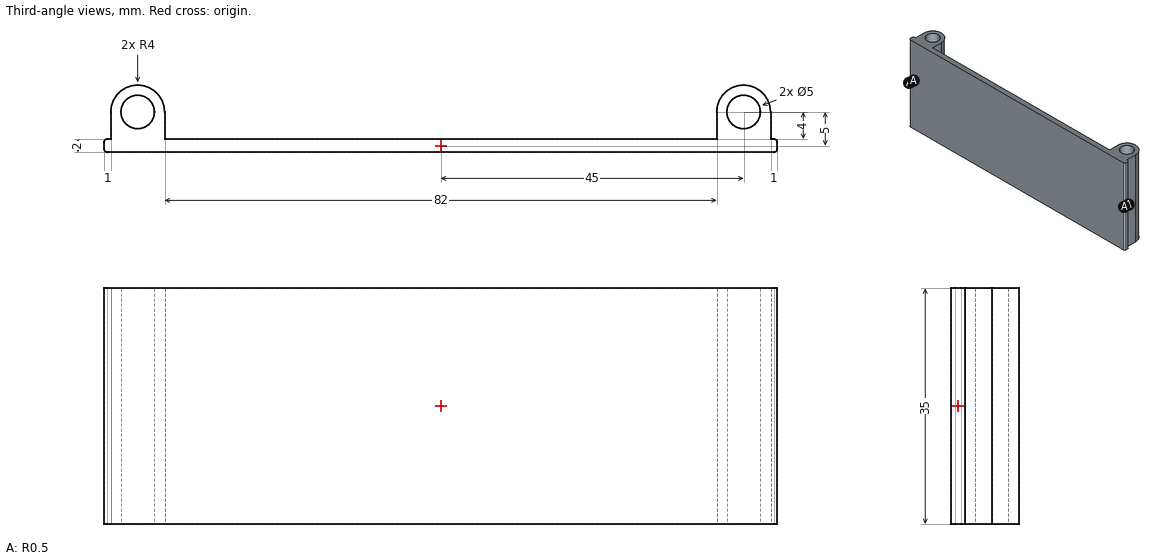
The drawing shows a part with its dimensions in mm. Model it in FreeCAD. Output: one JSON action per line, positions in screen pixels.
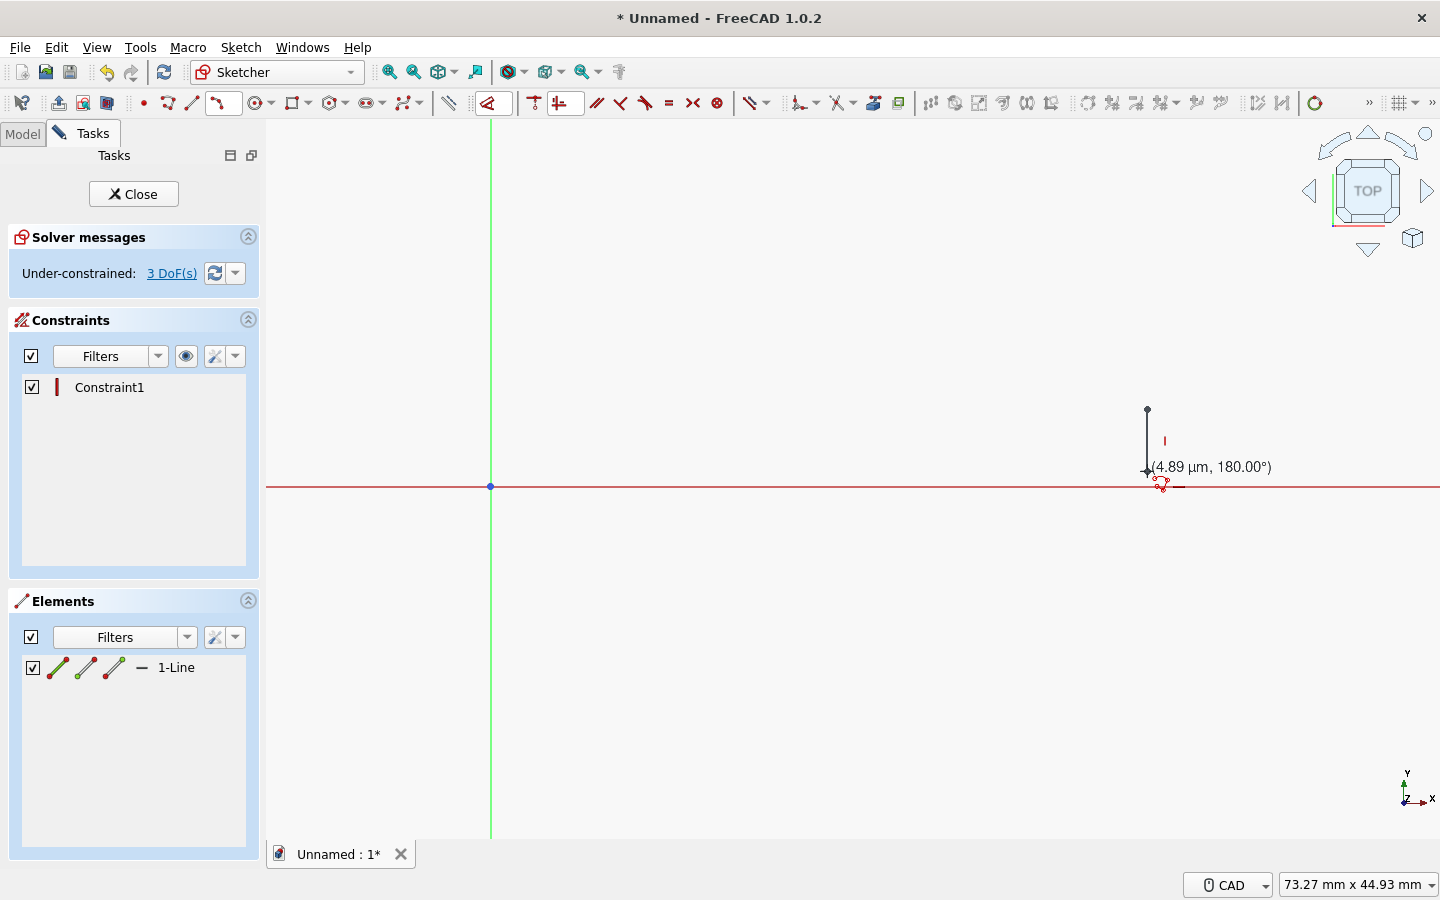
{"action": "scroll", "coordinate": [1024, 525], "scroll_direction": "down", "scroll_amount": 4}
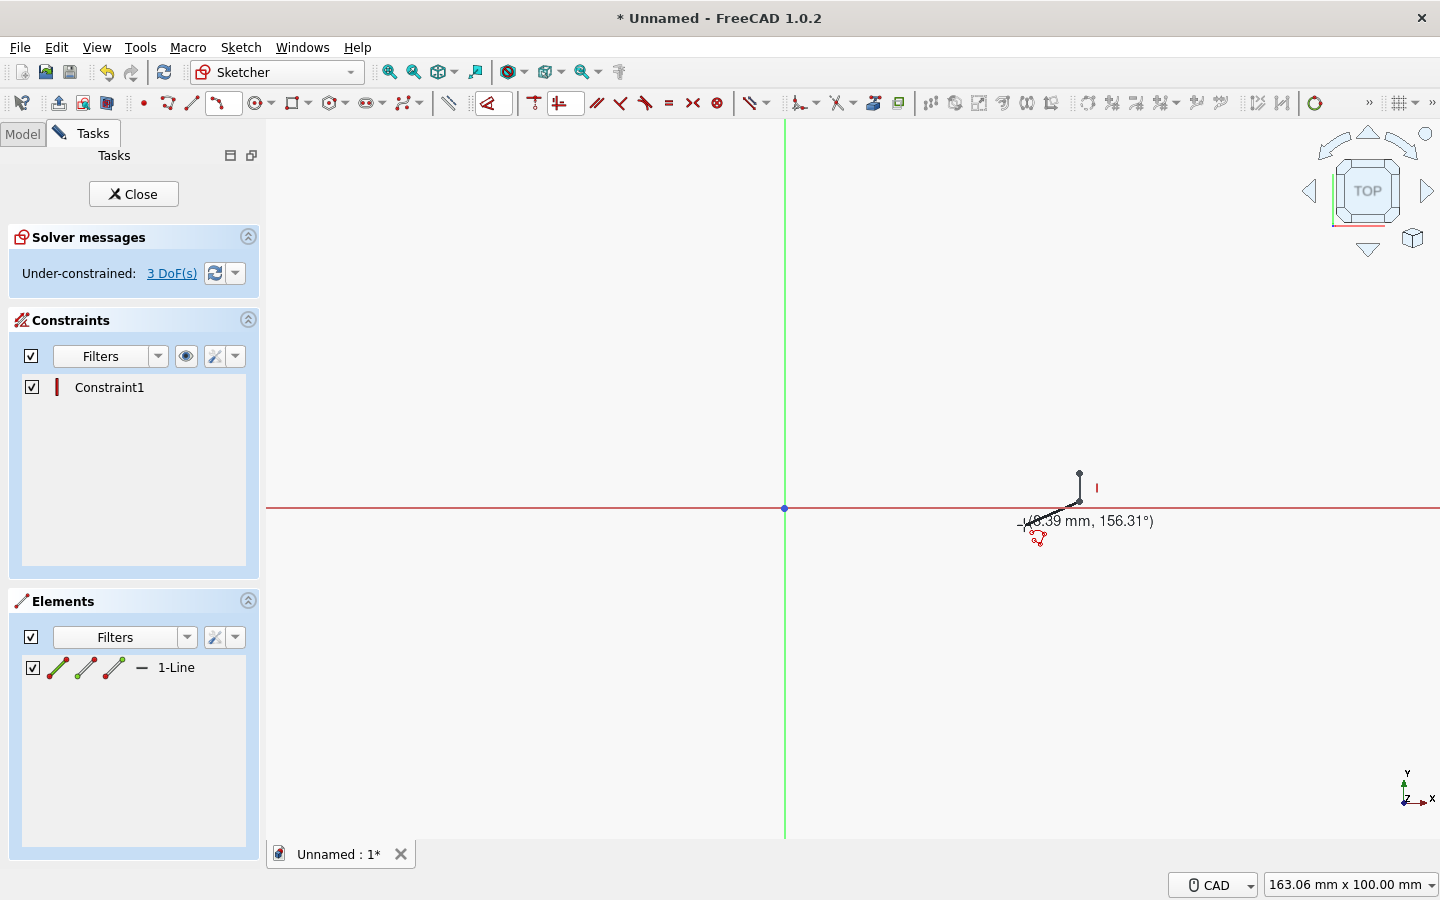
{"action": "scroll", "coordinate": [489, 501], "scroll_direction": "up", "scroll_amount": 4}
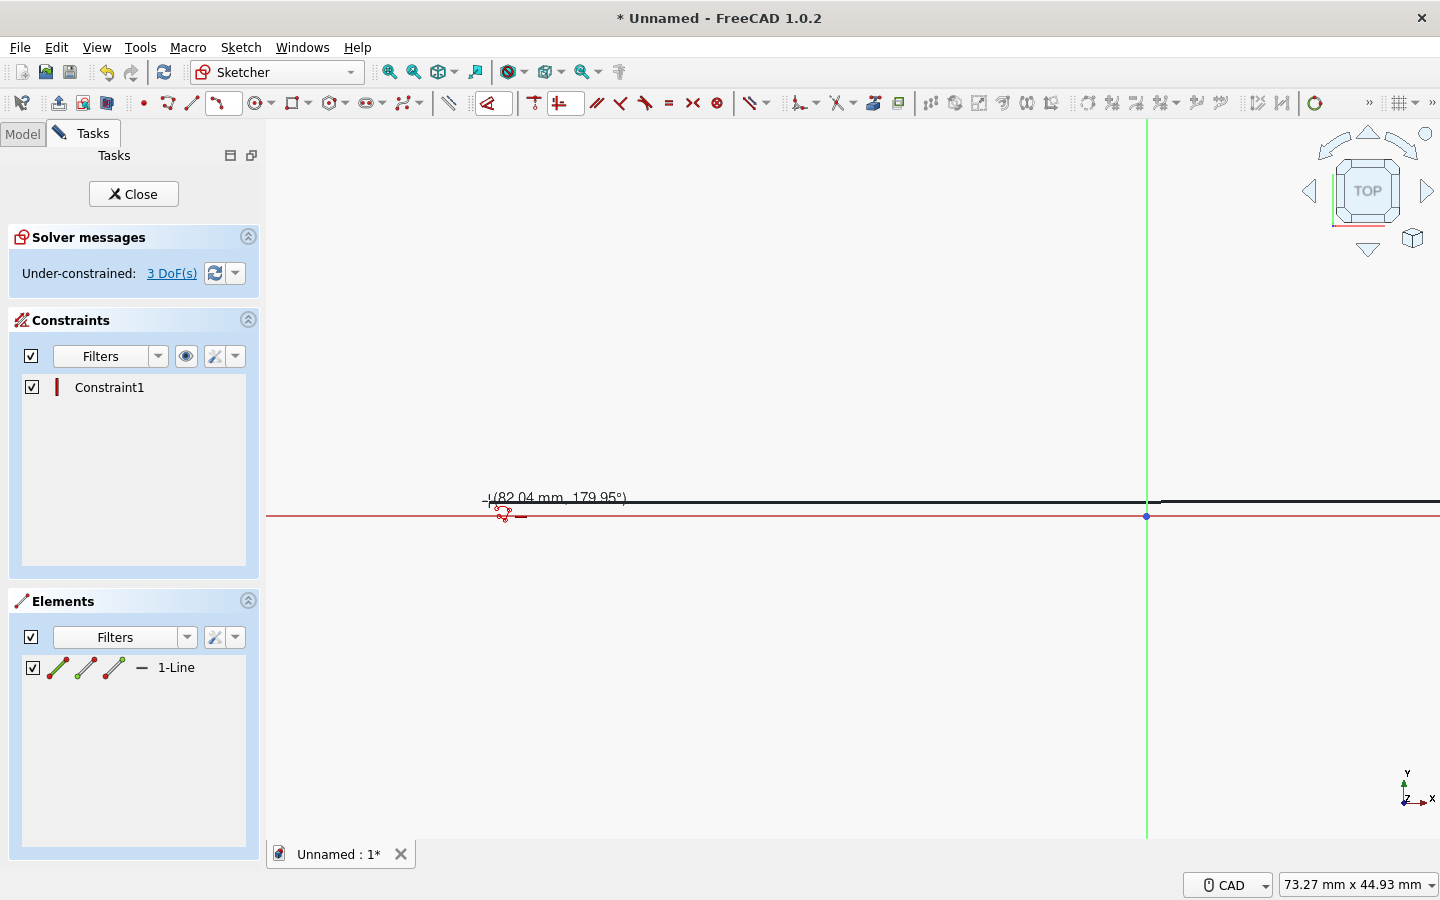
{"action": "left_click", "coordinate": [490, 500]}
{"action": "left_click", "coordinate": [490, 436]}
{"action": "right_click", "coordinate": [490, 436]}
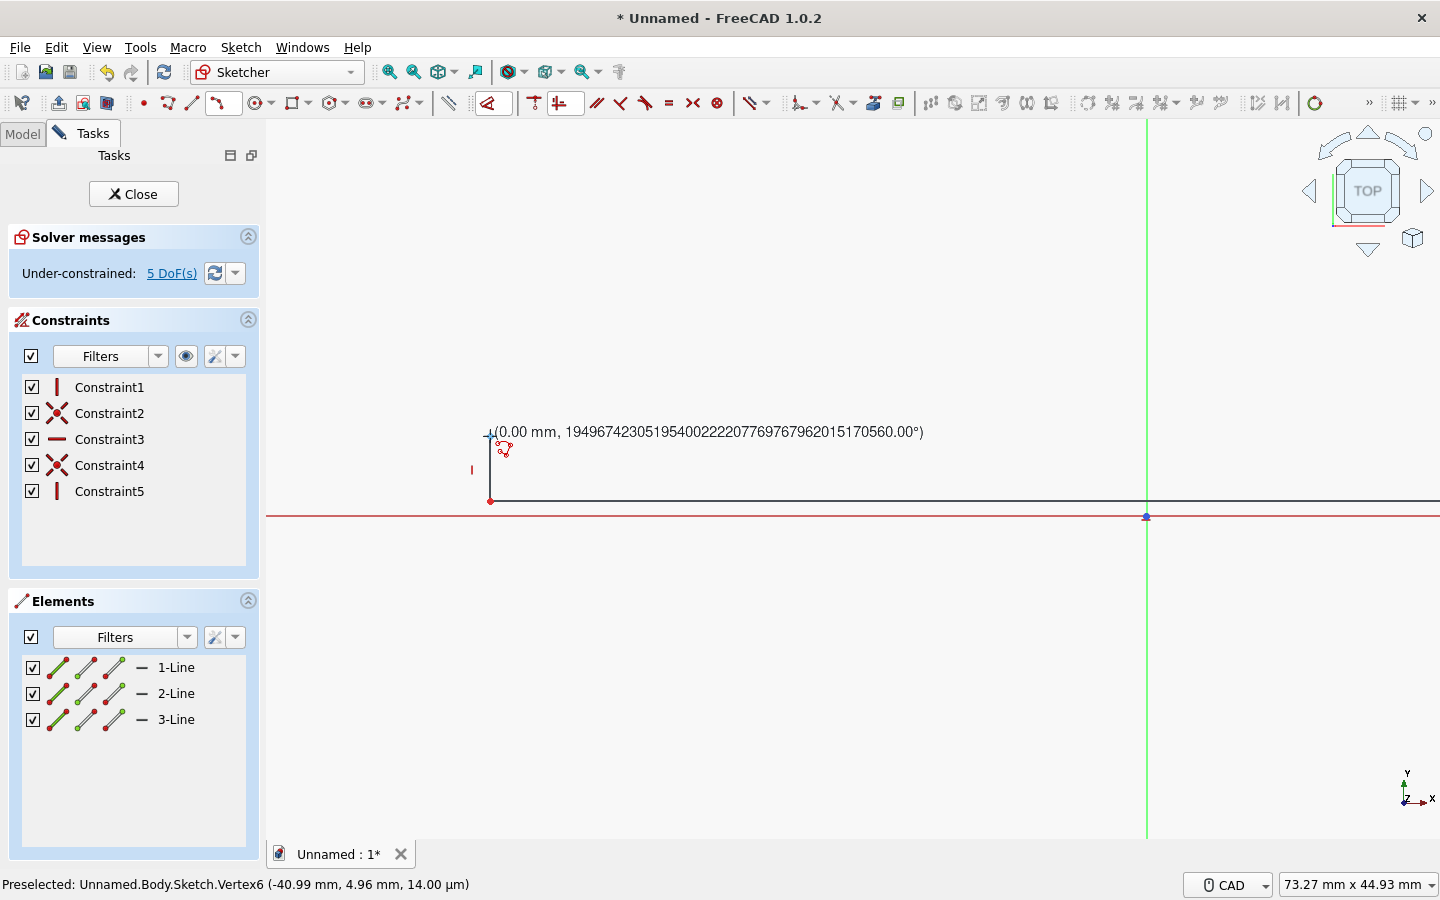
{"action": "left_click", "coordinate": [362, 436]}
{"action": "left_click", "coordinate": [362, 500]}
{"action": "left_click", "coordinate": [346, 500]}
{"action": "left_click", "coordinate": [346, 532]}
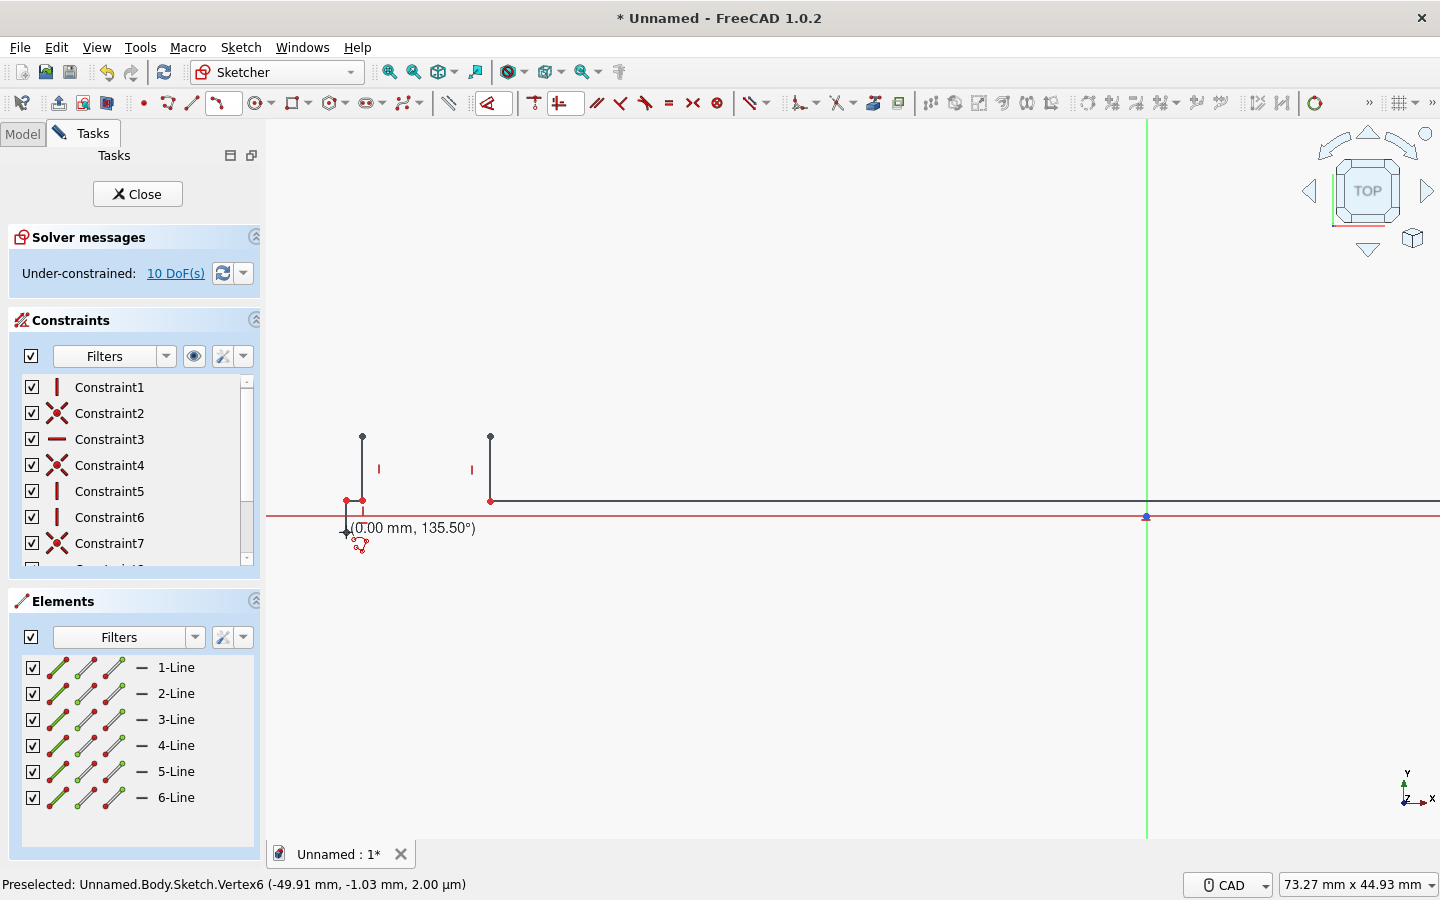
{"action": "scroll", "coordinate": [489, 501], "scroll_direction": "down", "scroll_amount": 4}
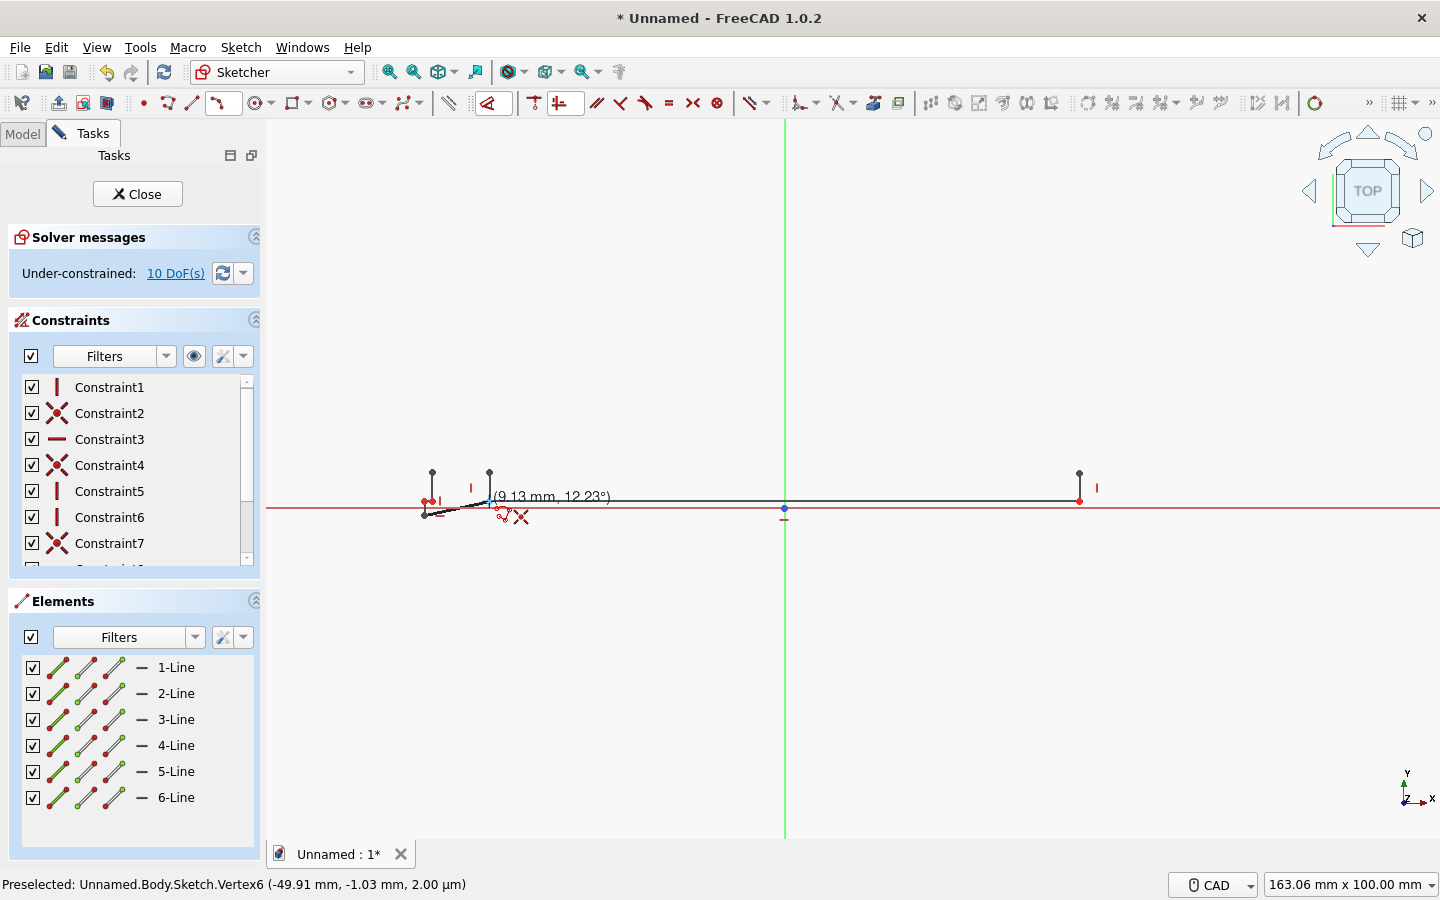
{"action": "scroll", "coordinate": [1145, 515], "scroll_direction": "up", "scroll_amount": 4}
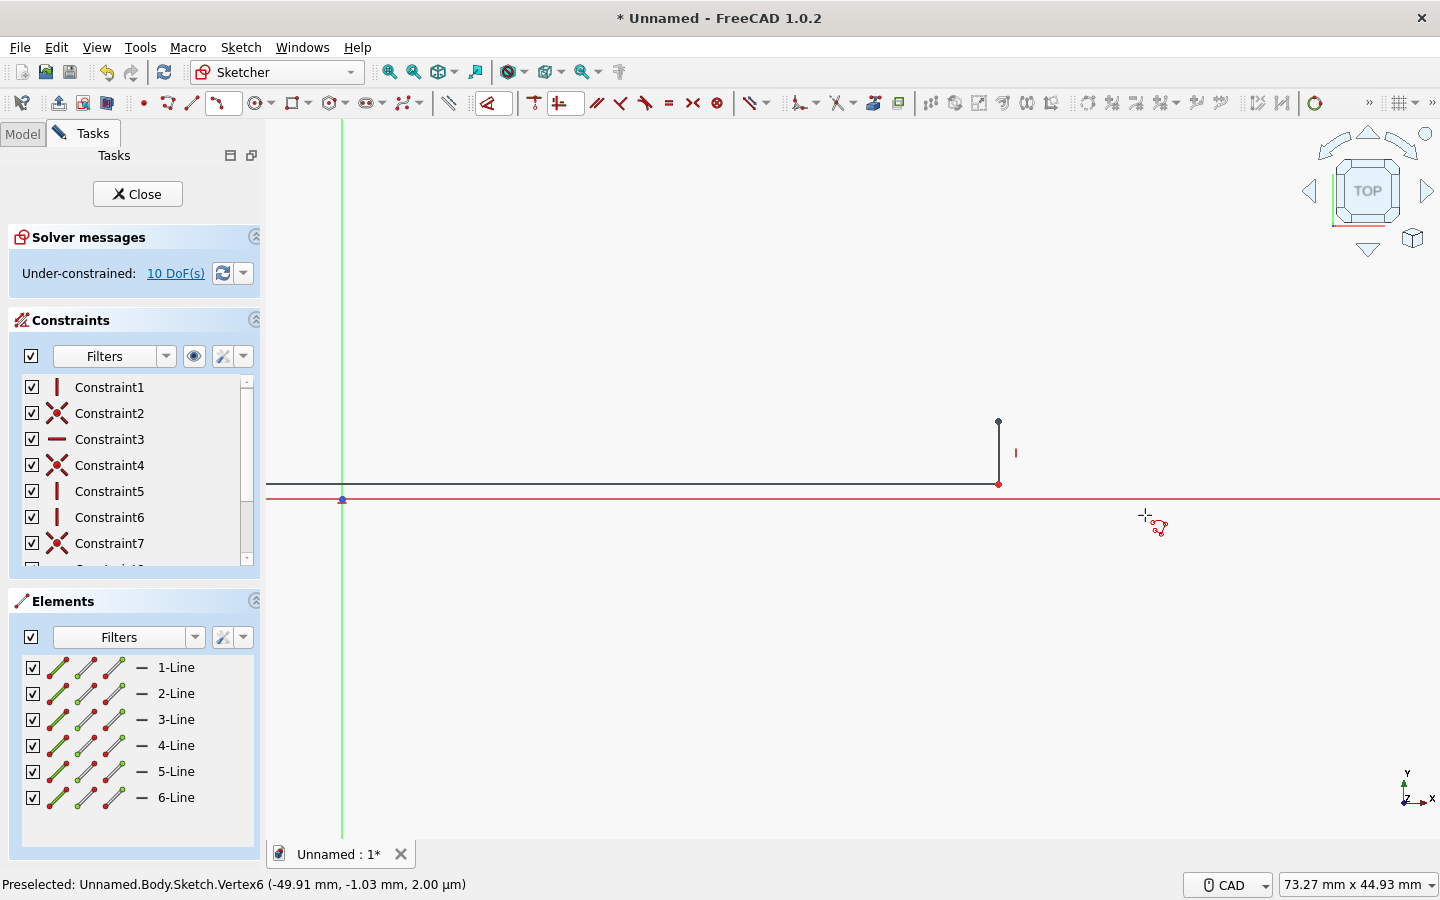
{"action": "left_click", "coordinate": [1143, 515]}
{"action": "left_click", "coordinate": [1143, 483]}
{"action": "left_click", "coordinate": [1127, 483]}
{"action": "left_click", "coordinate": [1127, 419]}
{"action": "right_click", "coordinate": [1127, 419]}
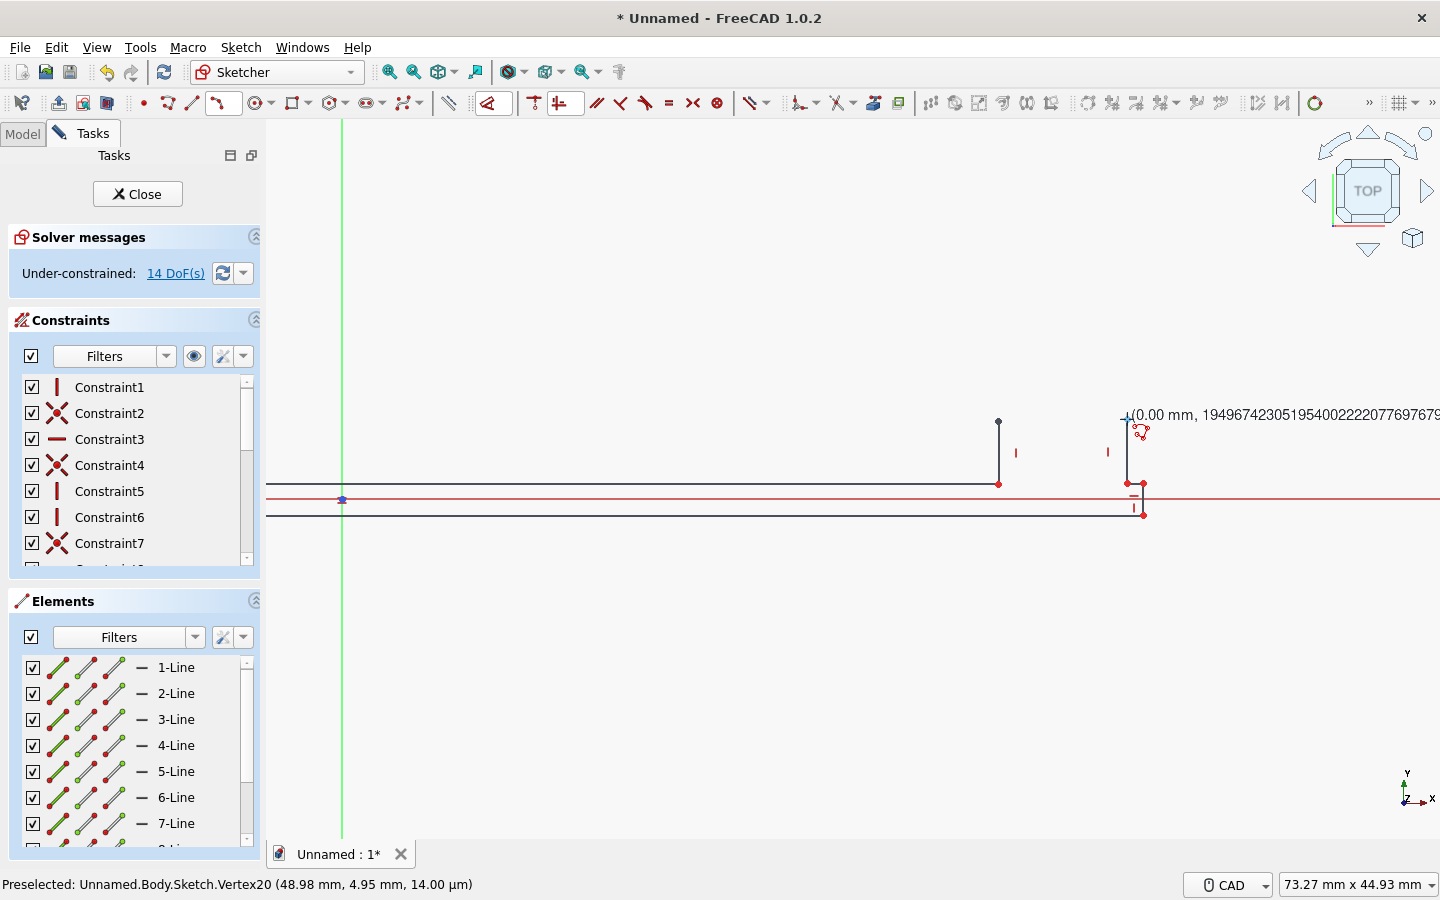
{"action": "left_click", "coordinate": [218, 104]}